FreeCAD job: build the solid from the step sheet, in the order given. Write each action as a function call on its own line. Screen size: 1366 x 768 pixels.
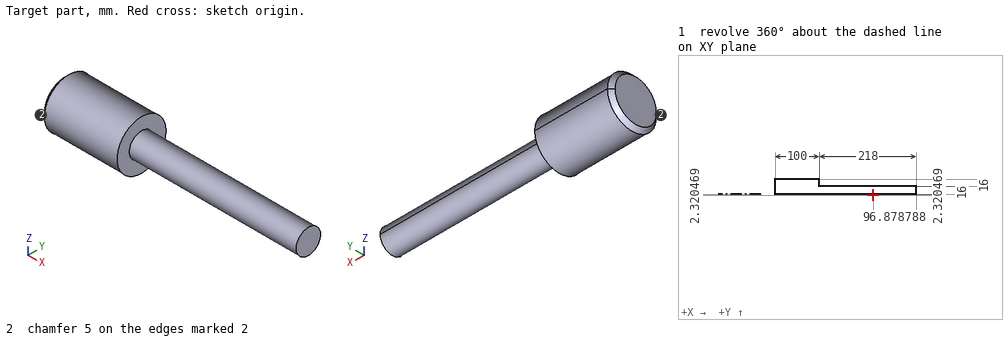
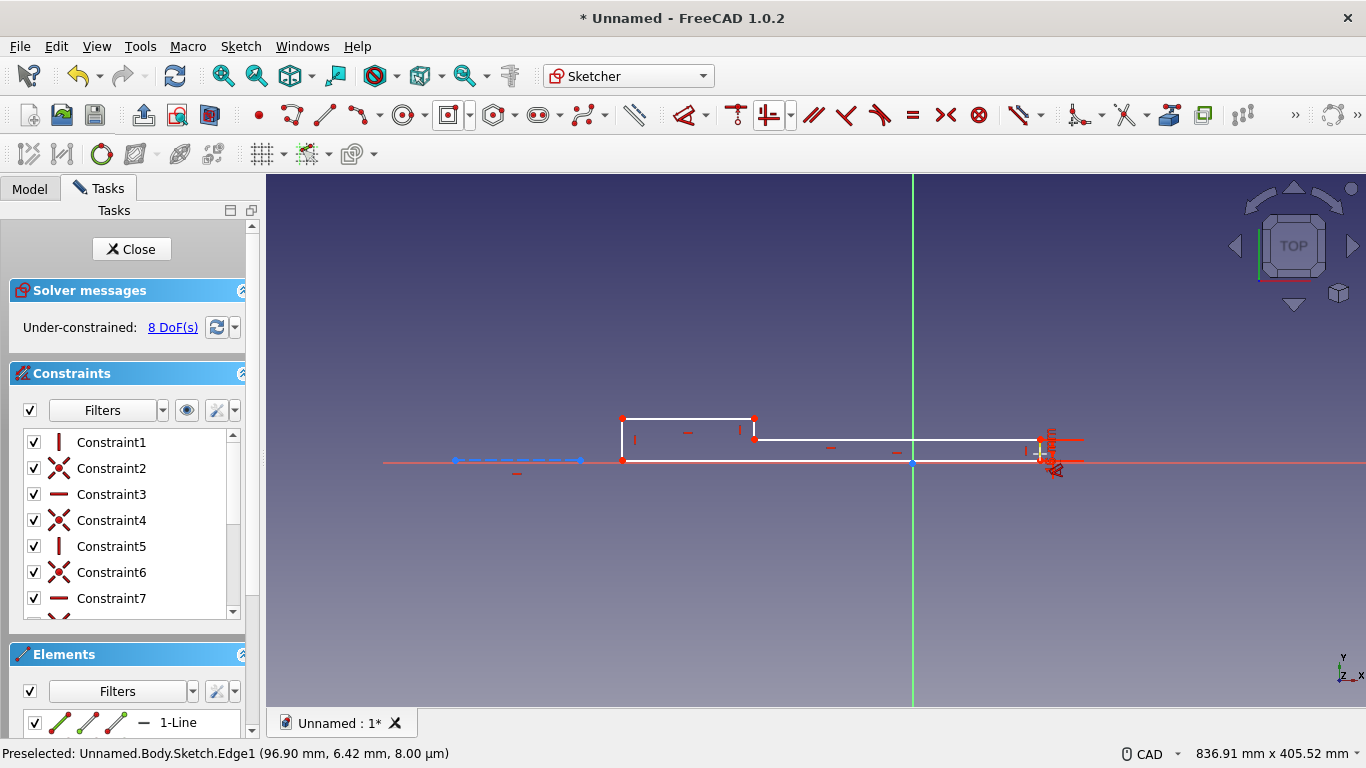
scroll(754, 433, up, 5)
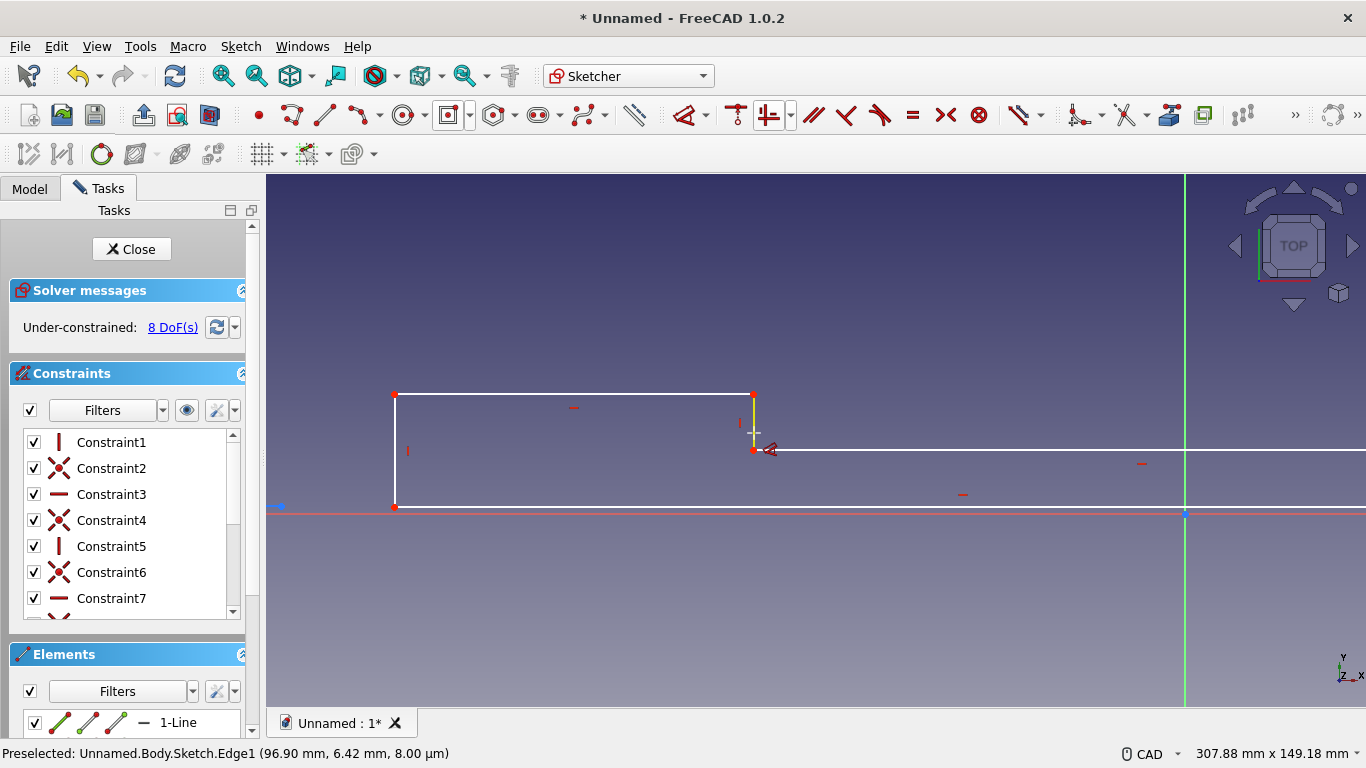
click(754, 433)
click(788, 422)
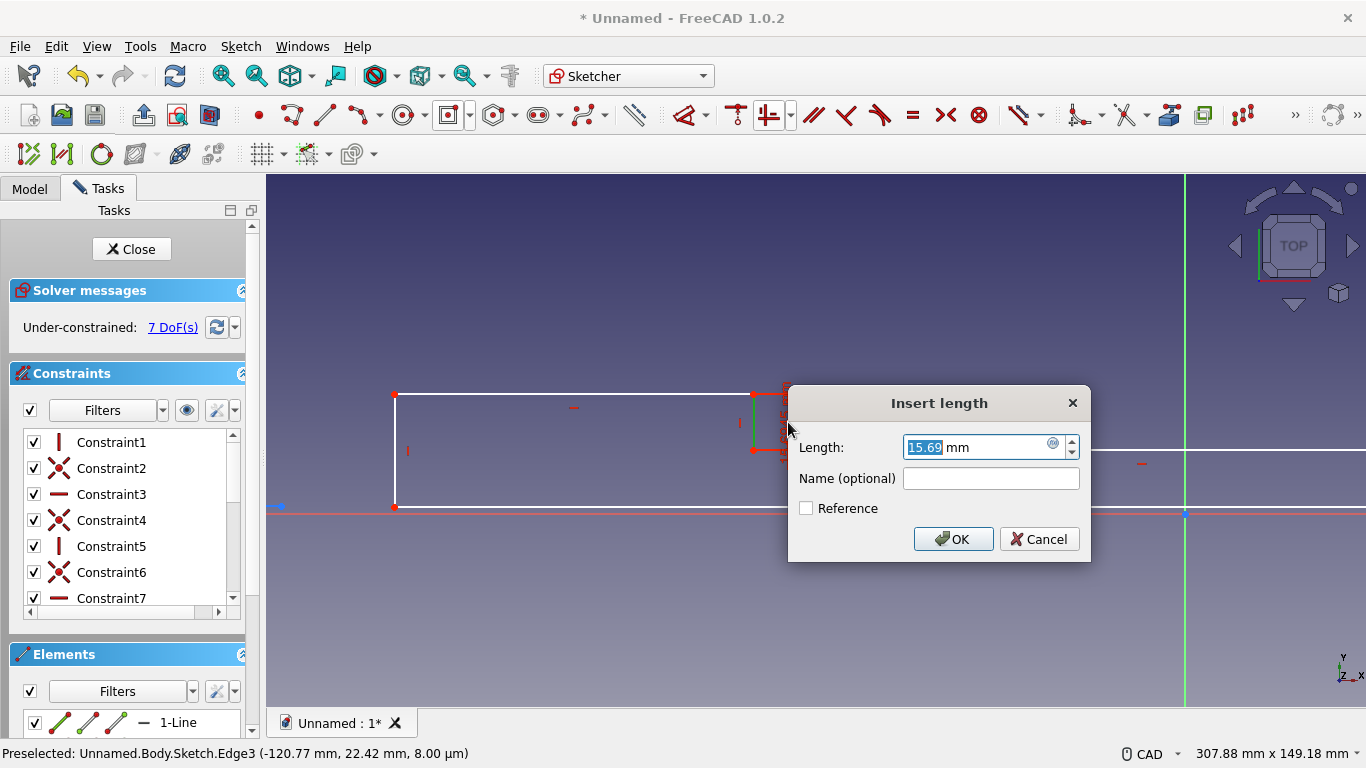
text(16)
key(Return)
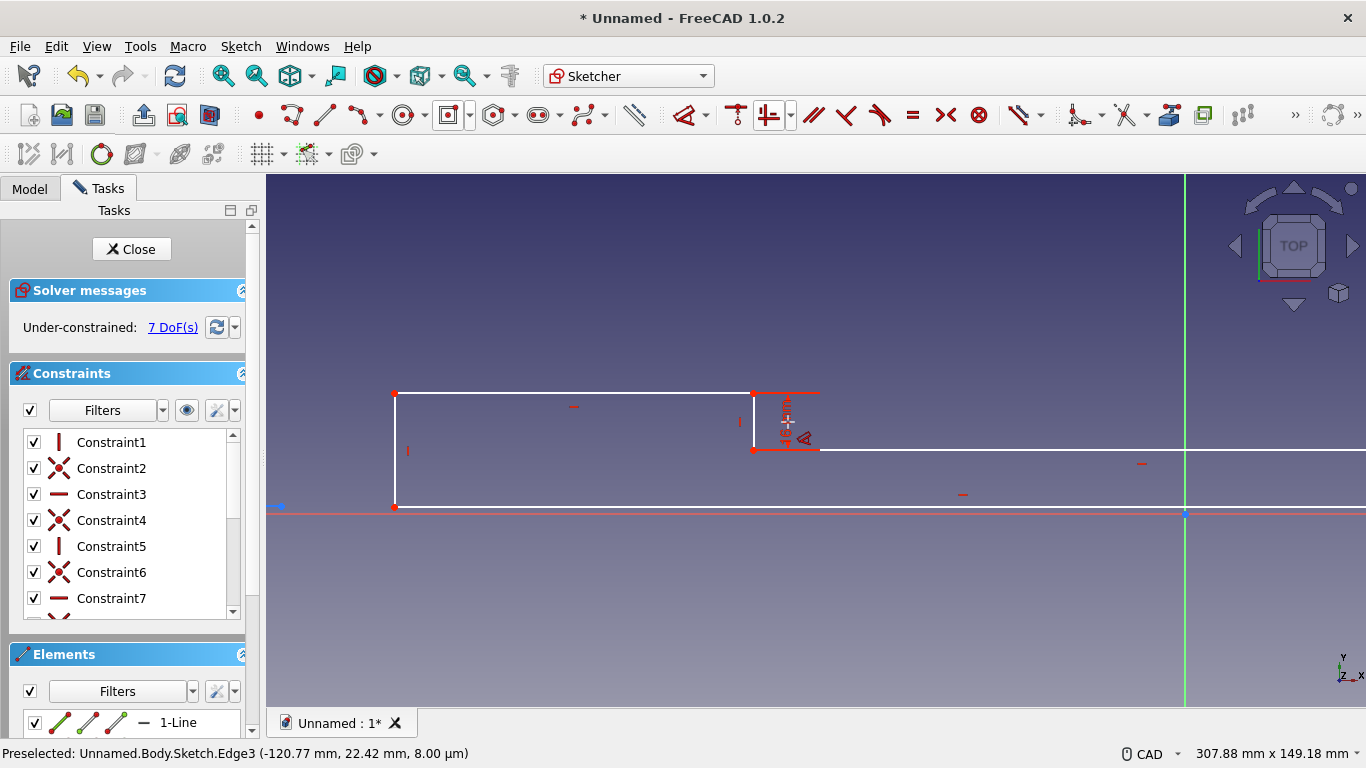
click(987, 450)
click(977, 416)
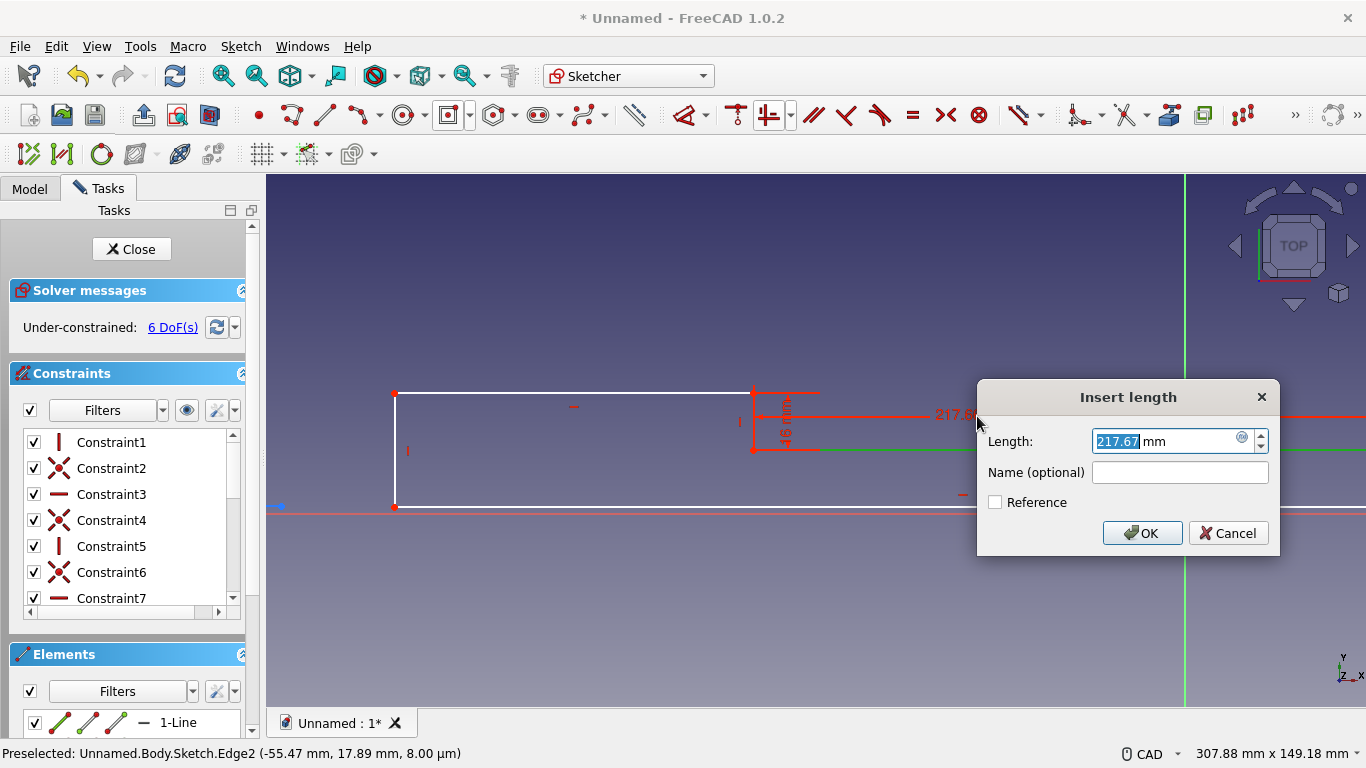
text(218)
key(Return)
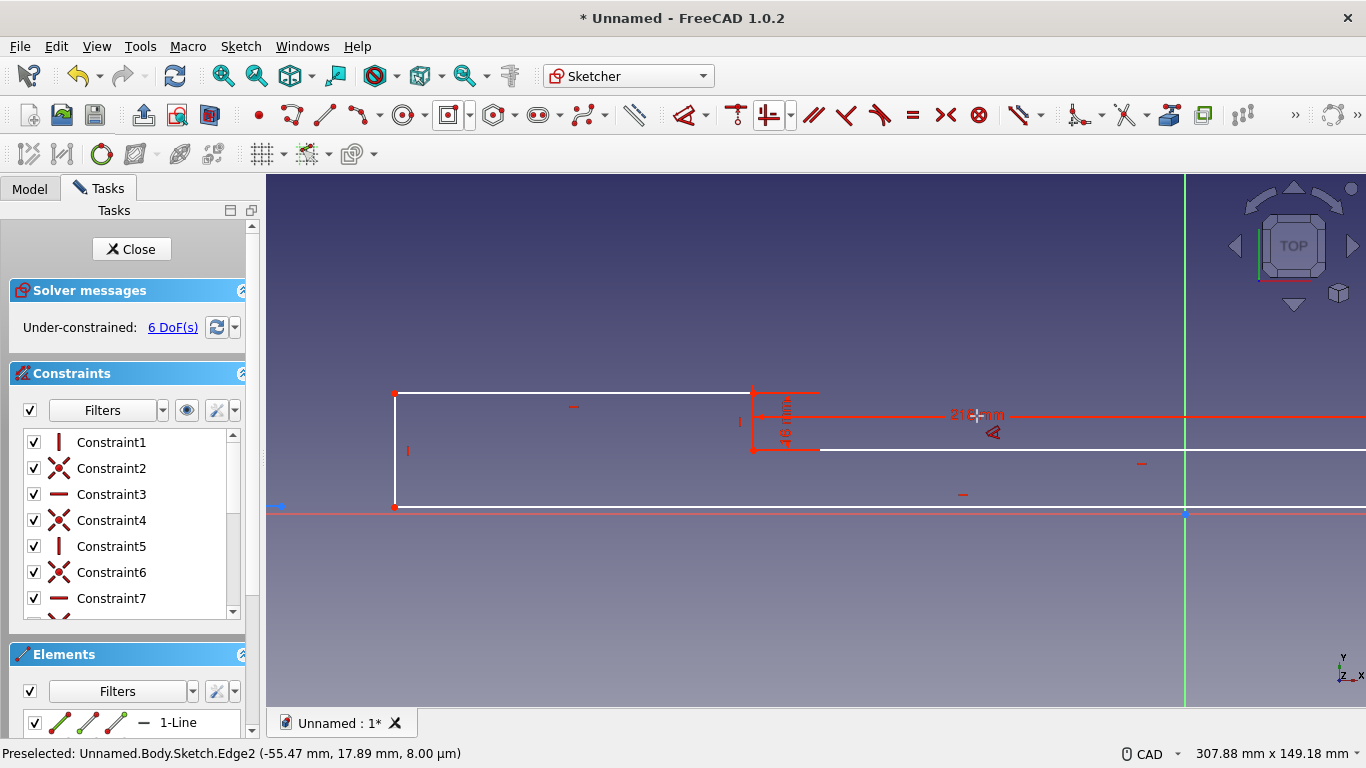
click(646, 393)
click(574, 359)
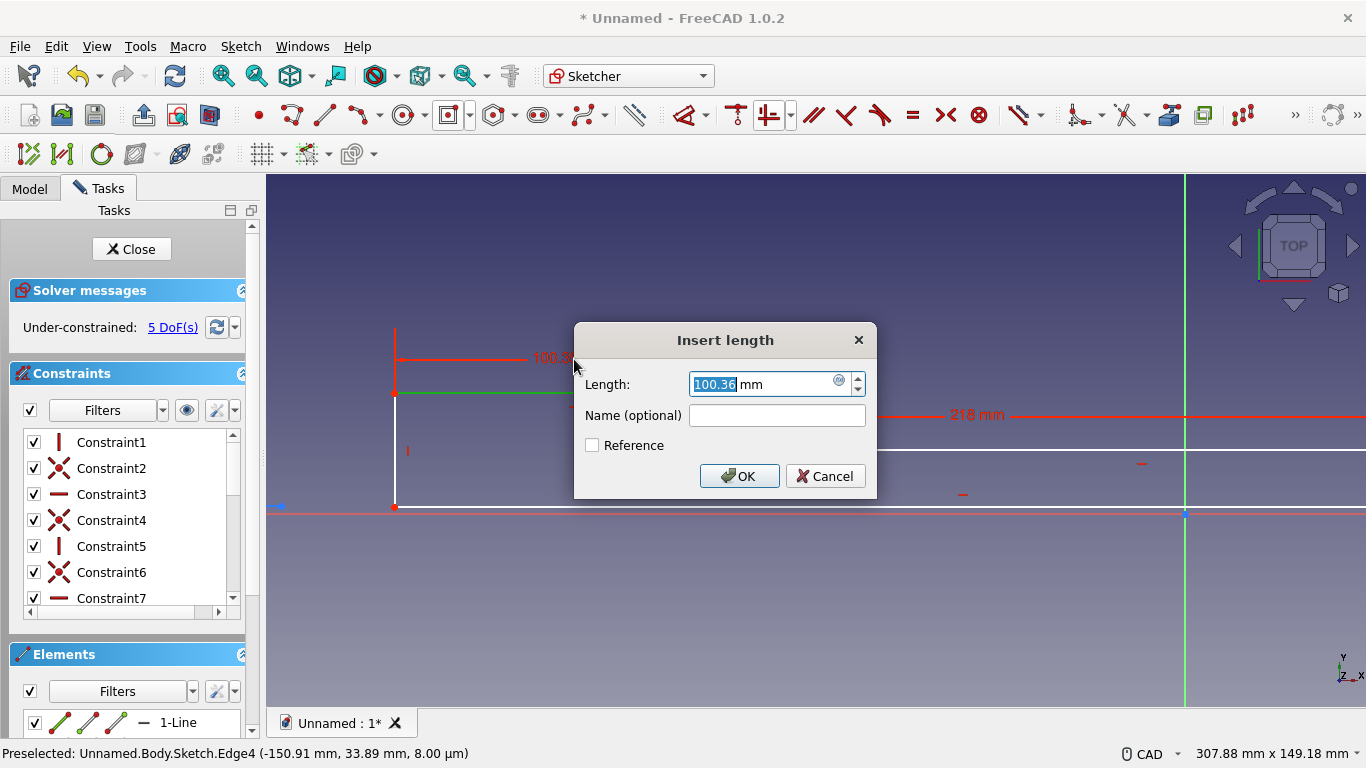
text(100)
key(Return)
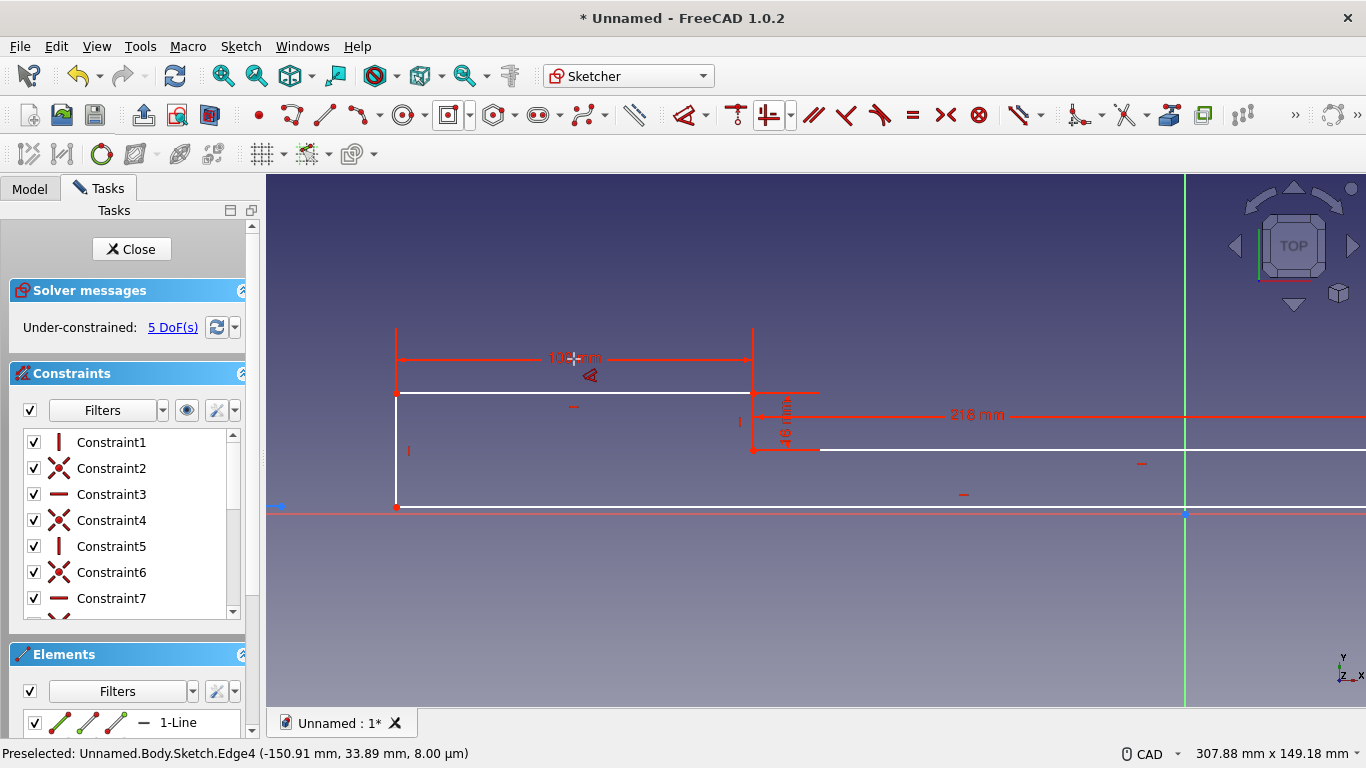
scroll(754, 433, down, 5)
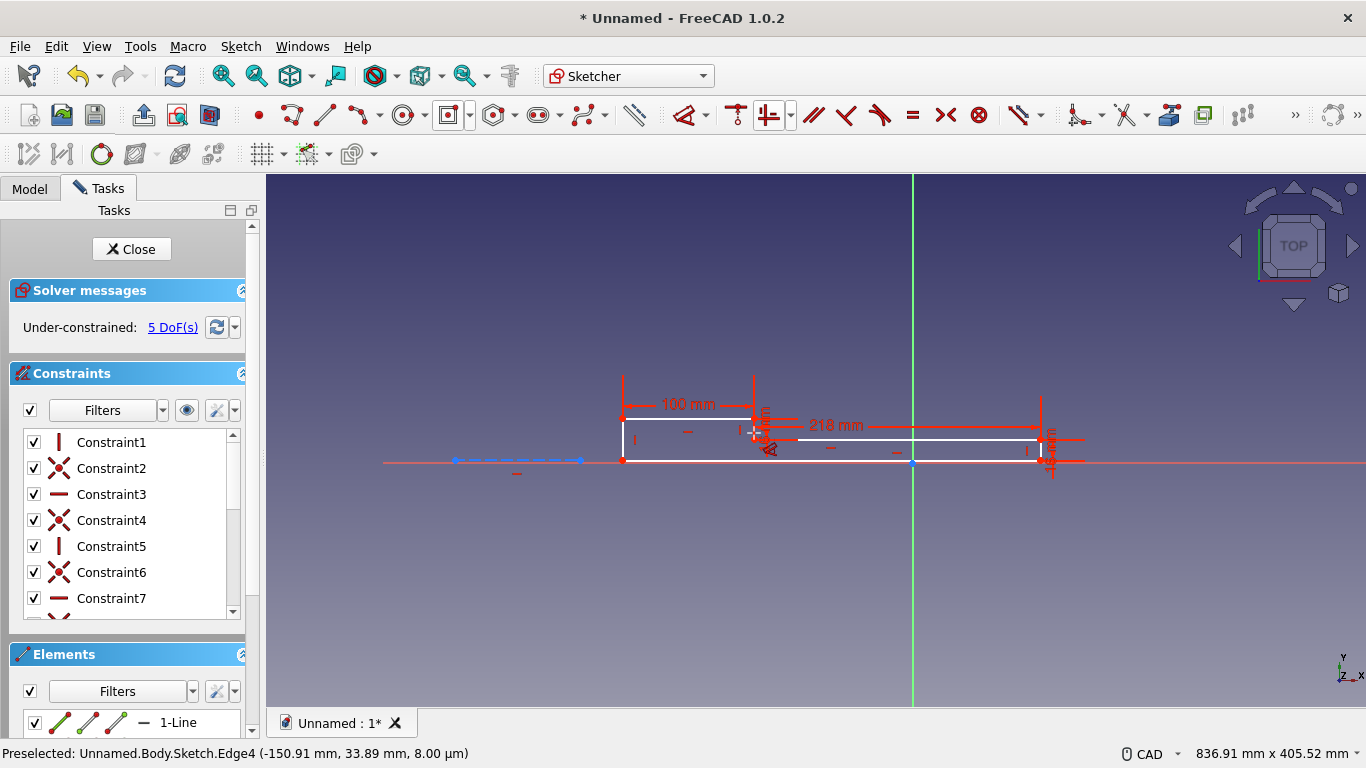
scroll(1041, 461, up, 13)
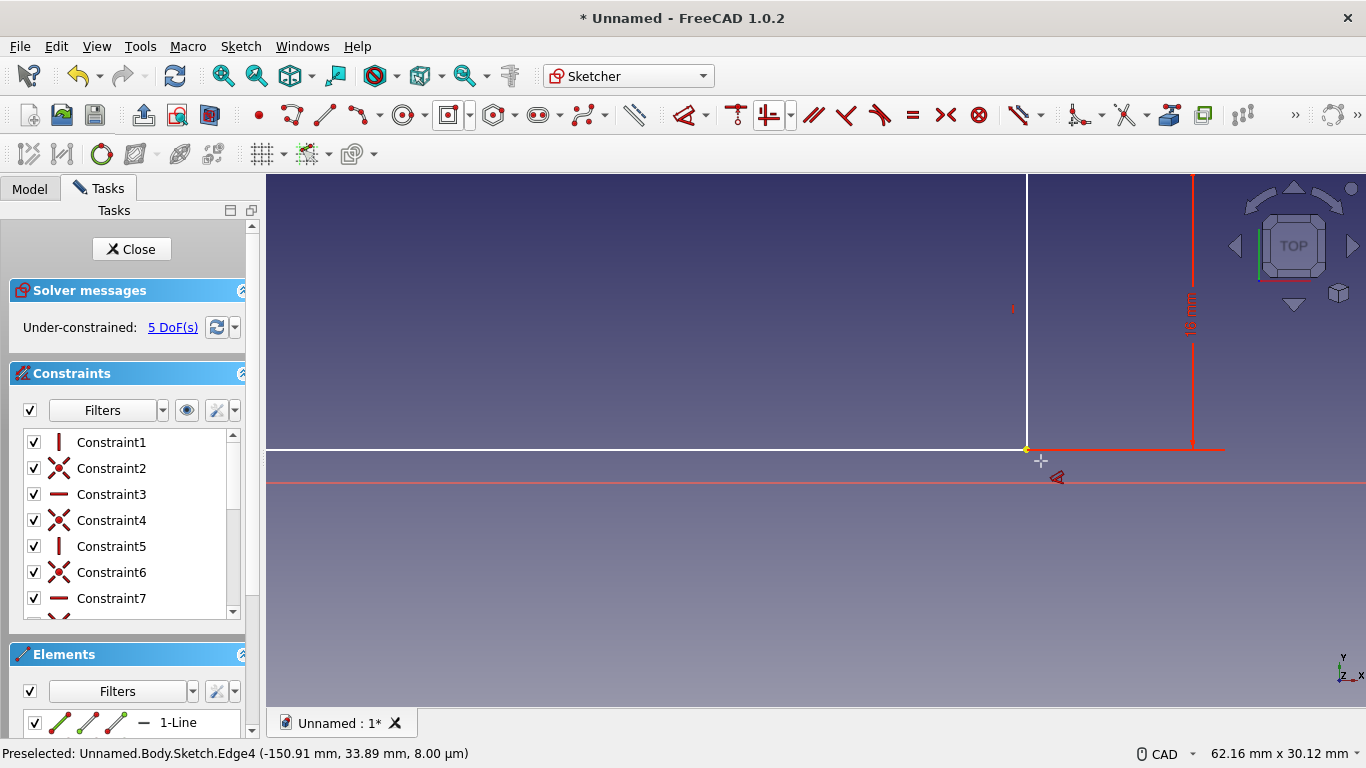
click(1027, 450)
click(1061, 466)